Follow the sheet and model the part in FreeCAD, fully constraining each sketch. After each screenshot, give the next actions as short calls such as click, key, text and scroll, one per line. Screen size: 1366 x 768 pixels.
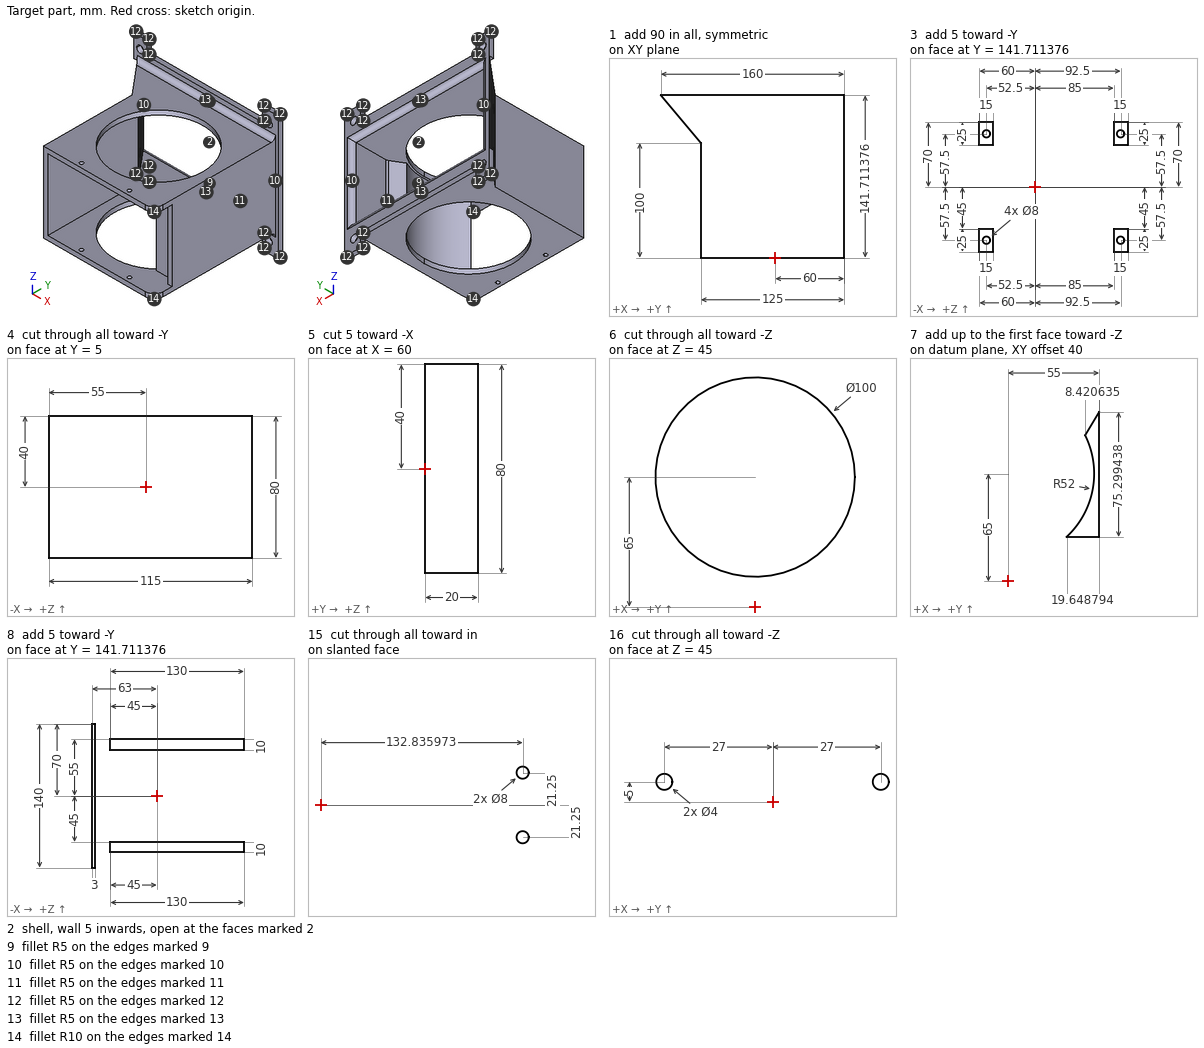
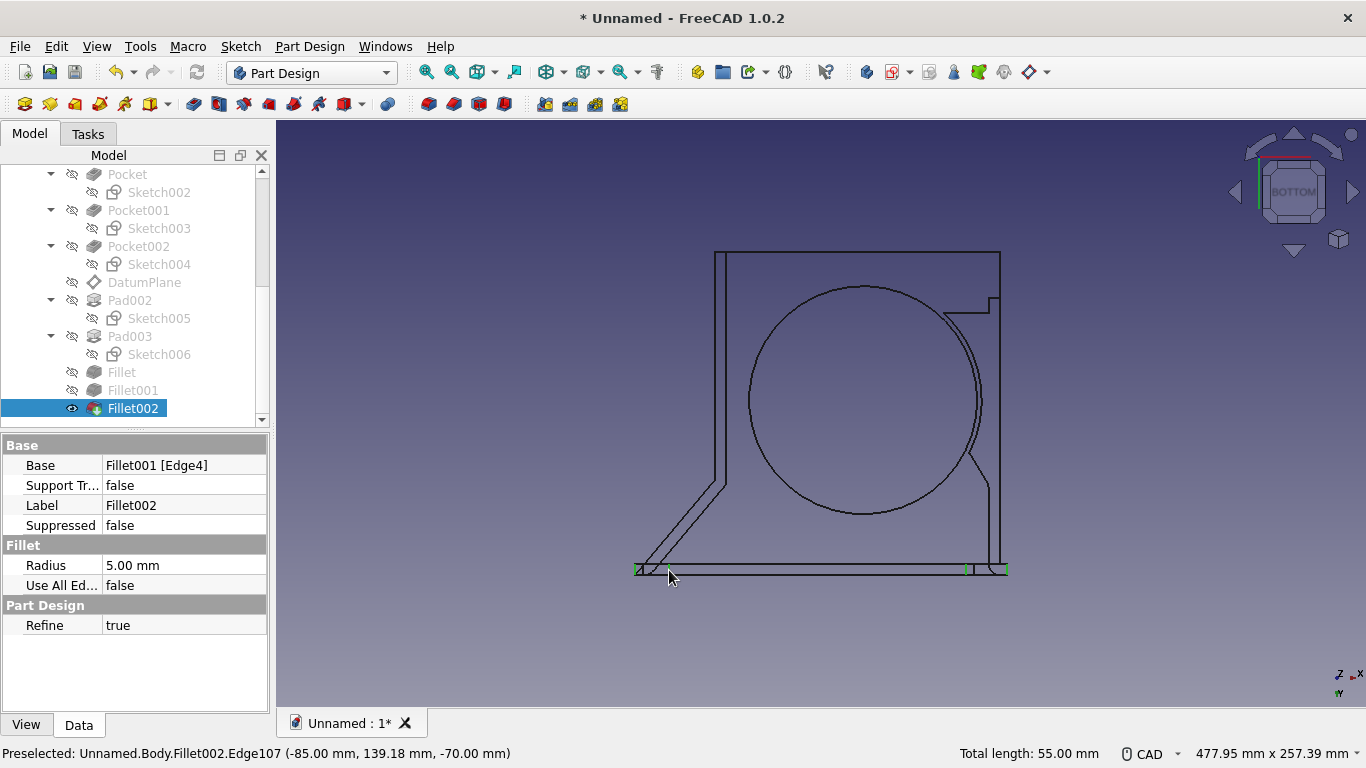
key(4)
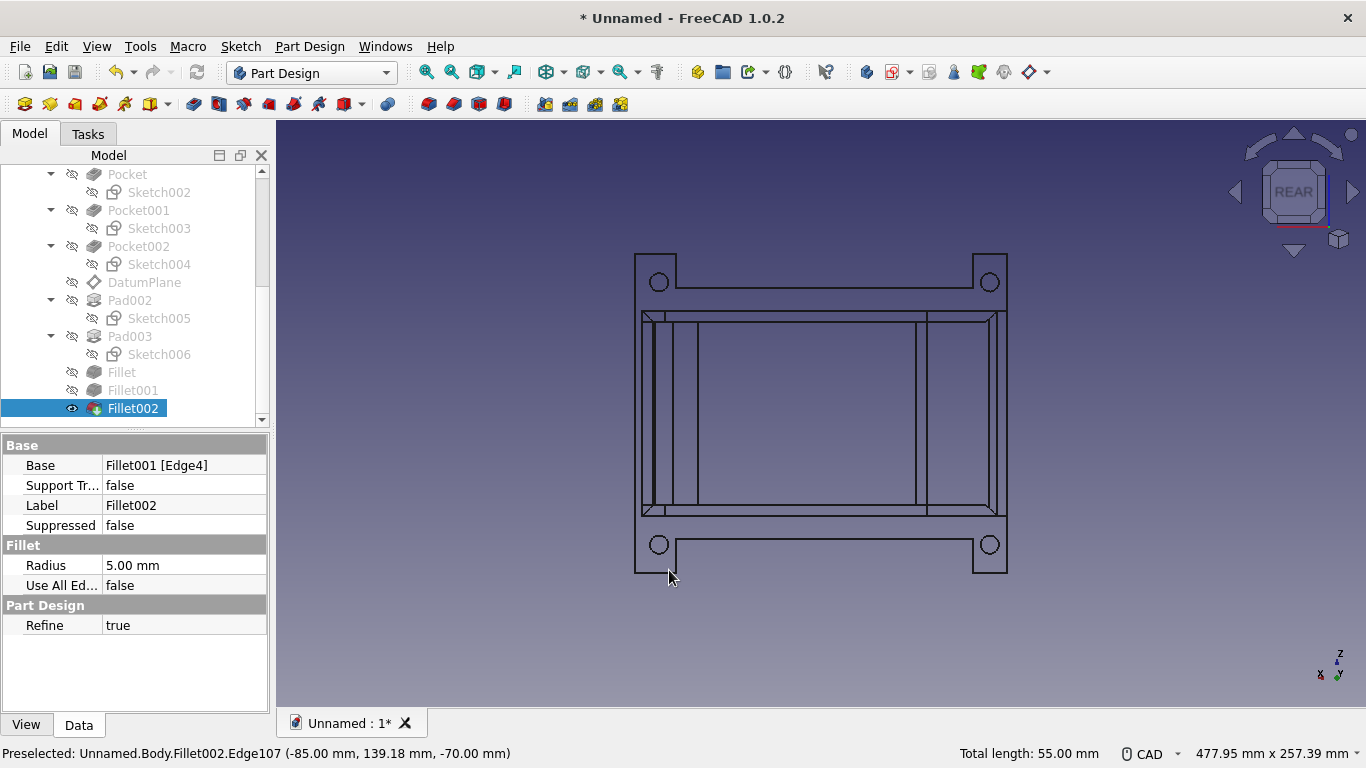
scroll(973, 287, up, 7)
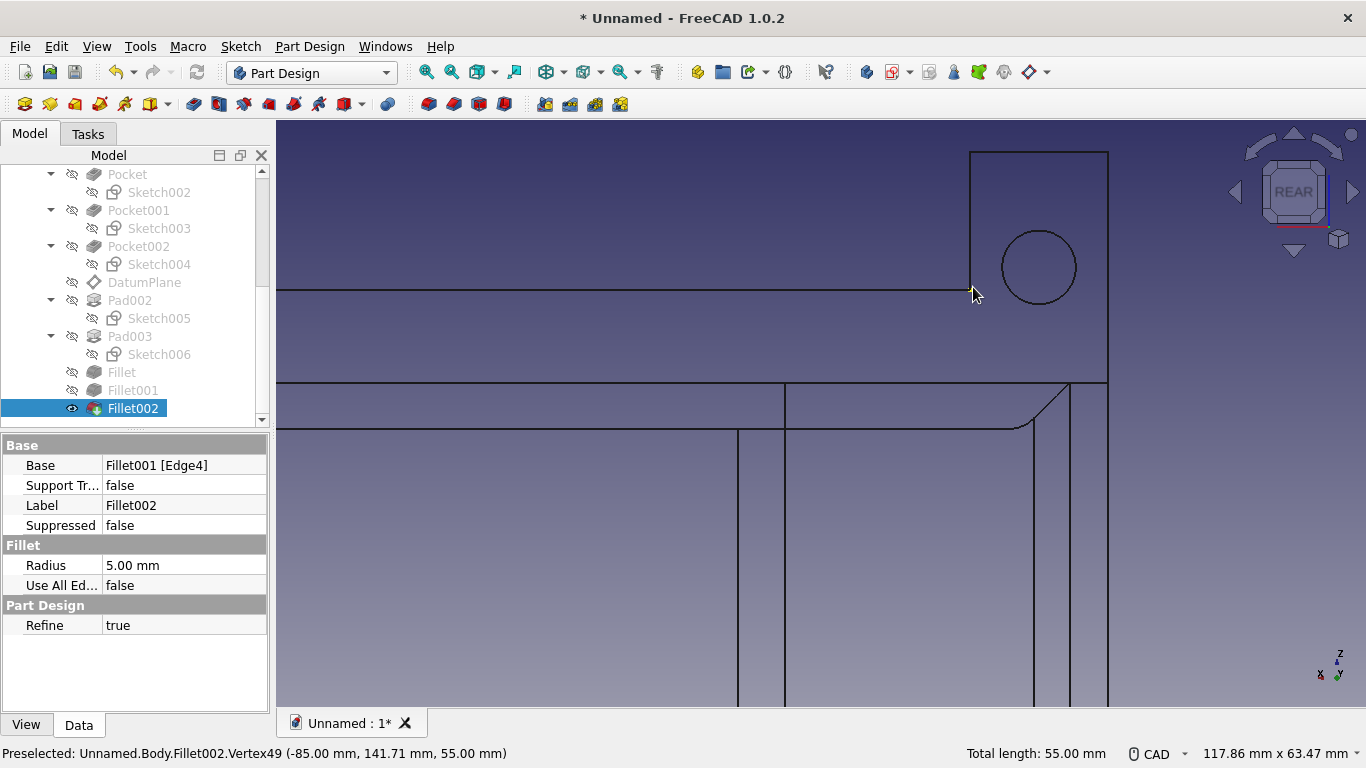
key(v)
key(f)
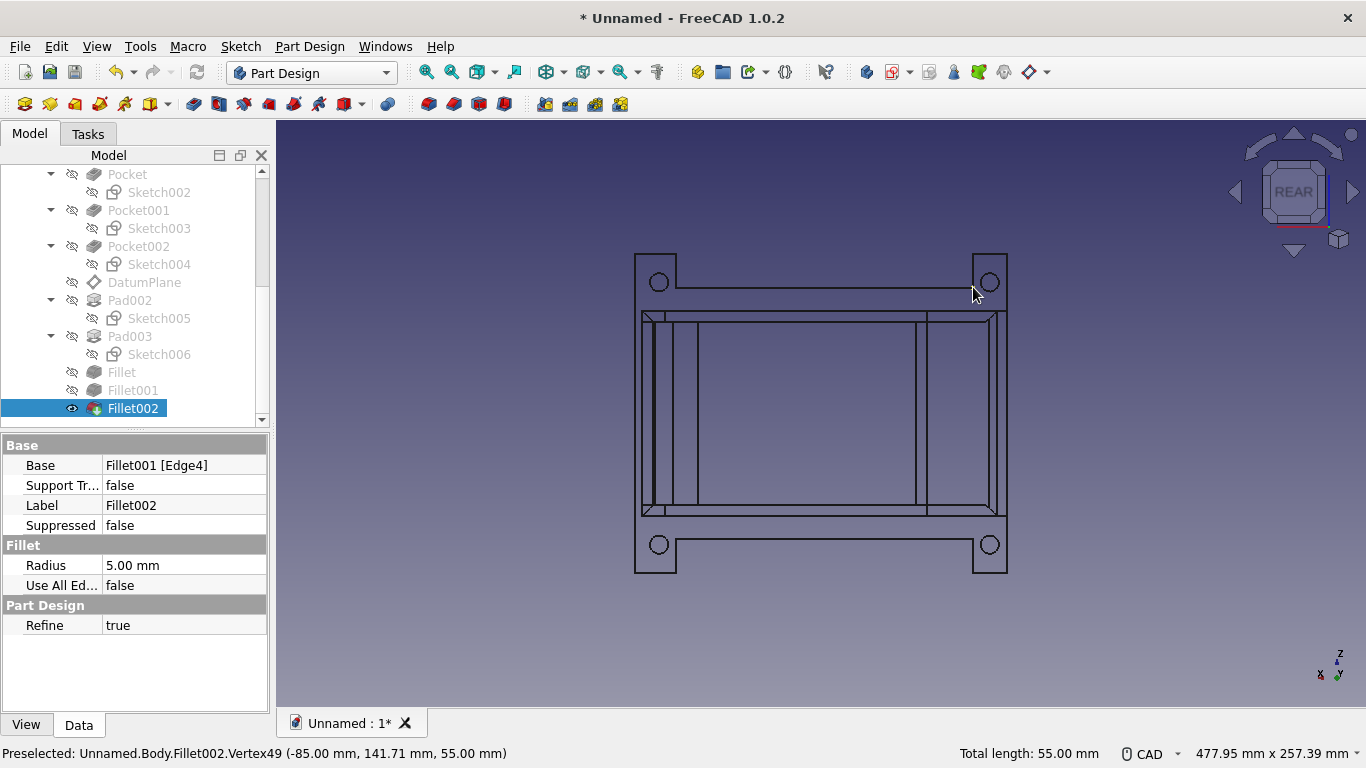
key(6)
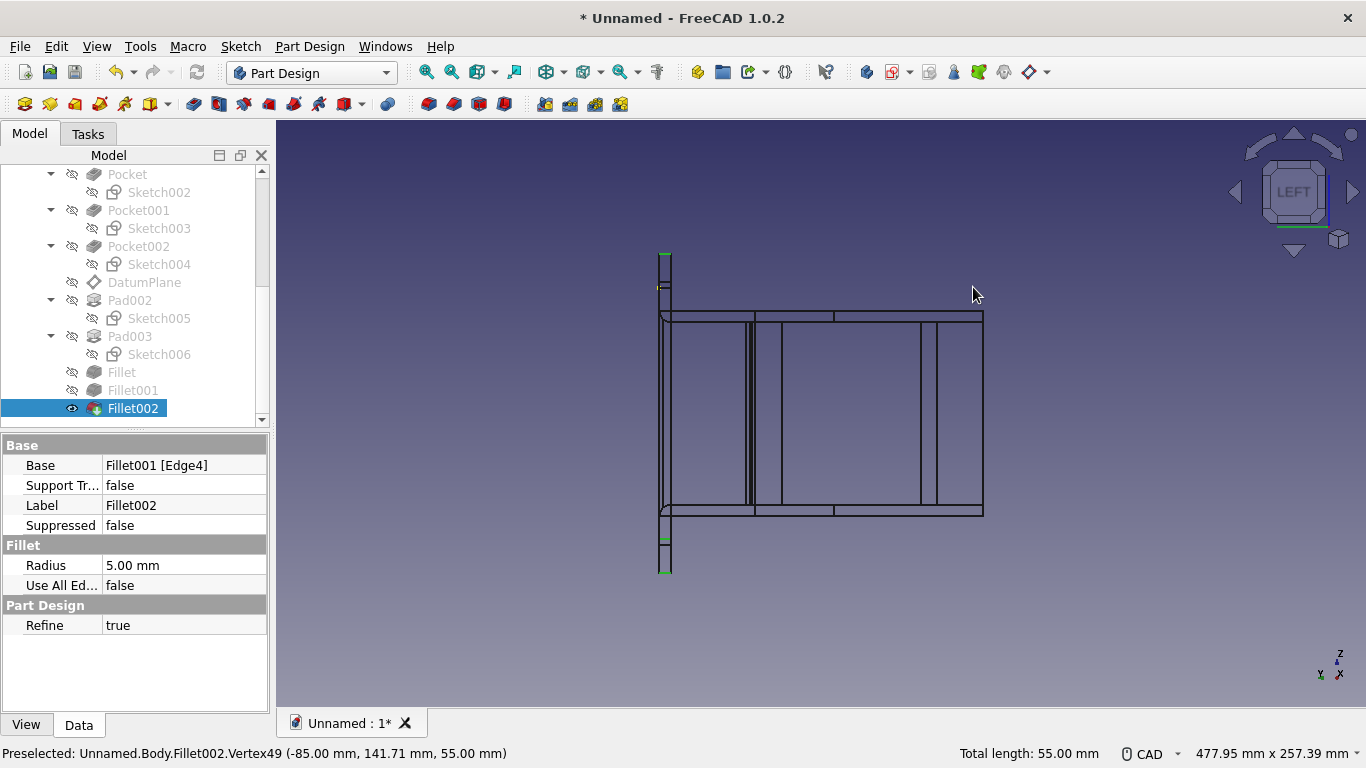
scroll(665, 287, up, 7)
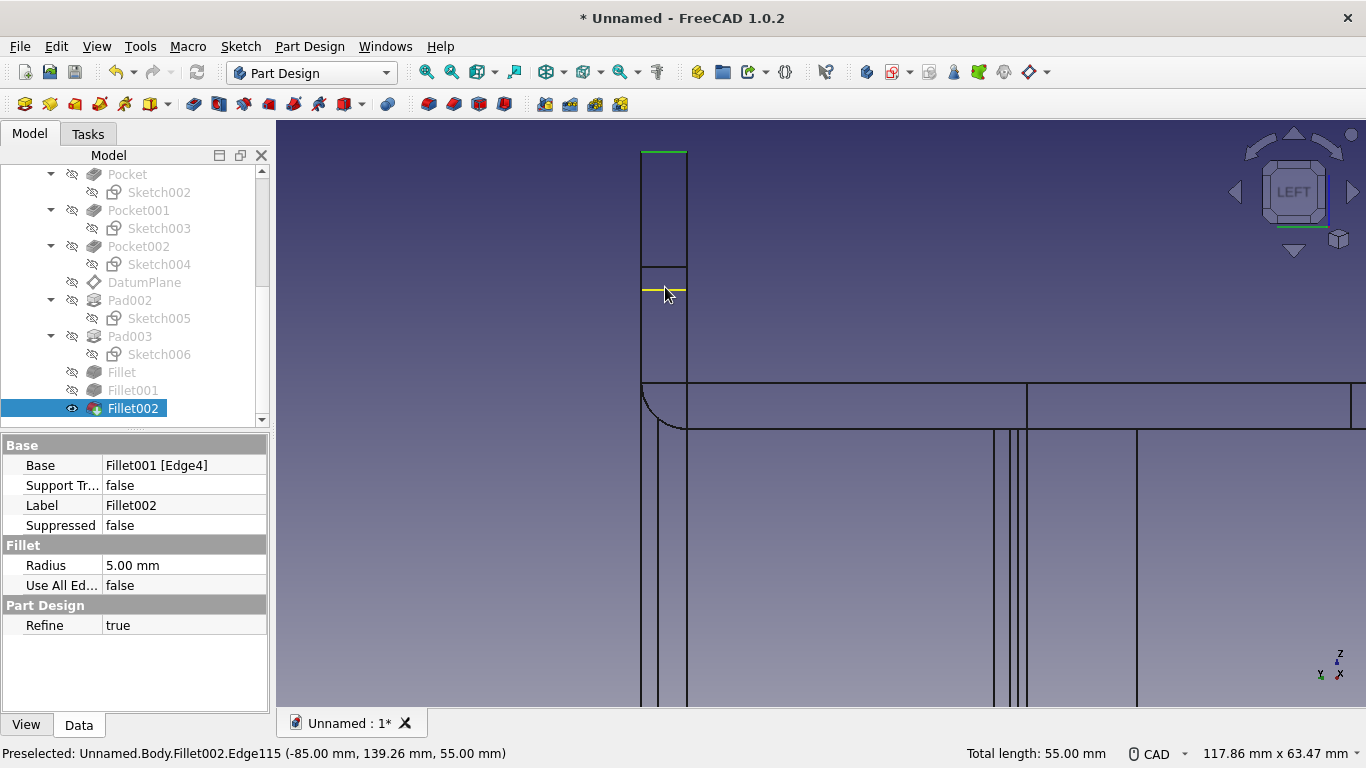
click(664, 289, ctrl)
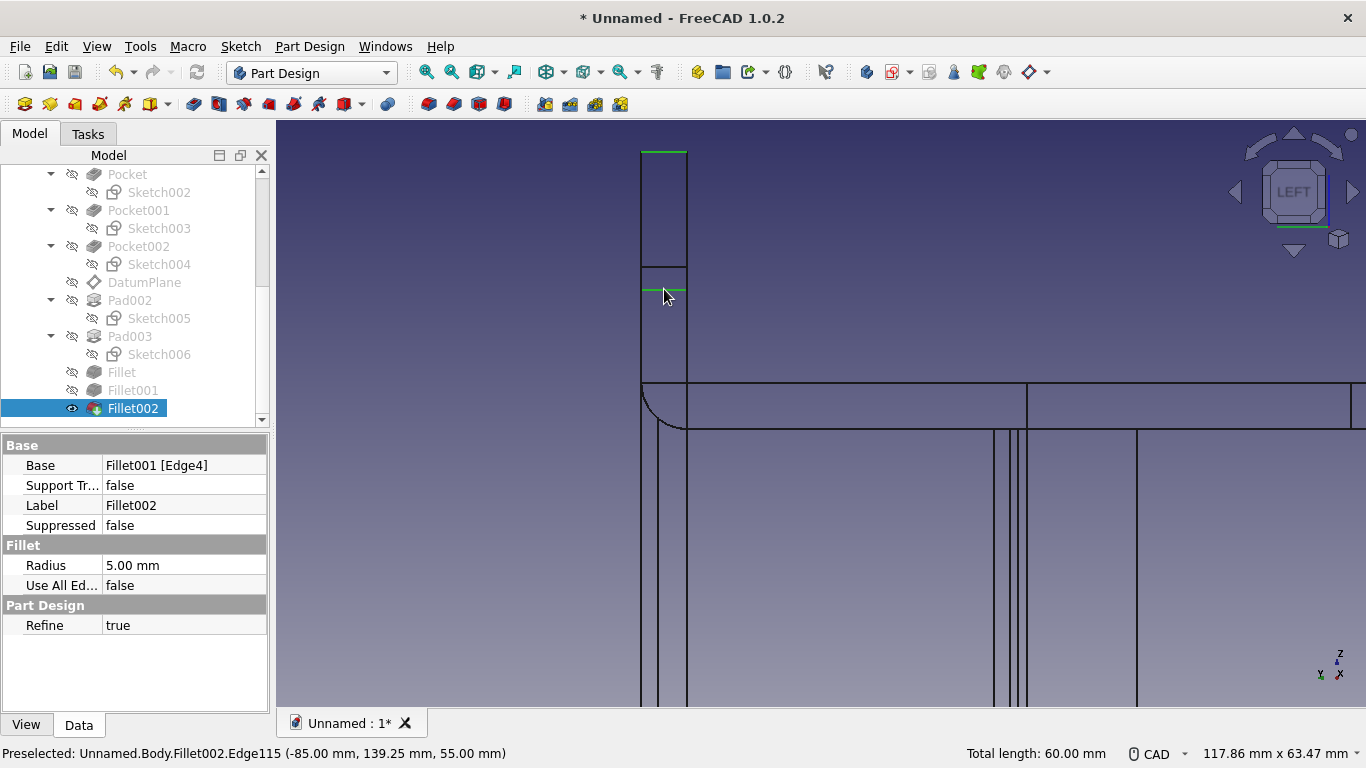
key(v)
key(1)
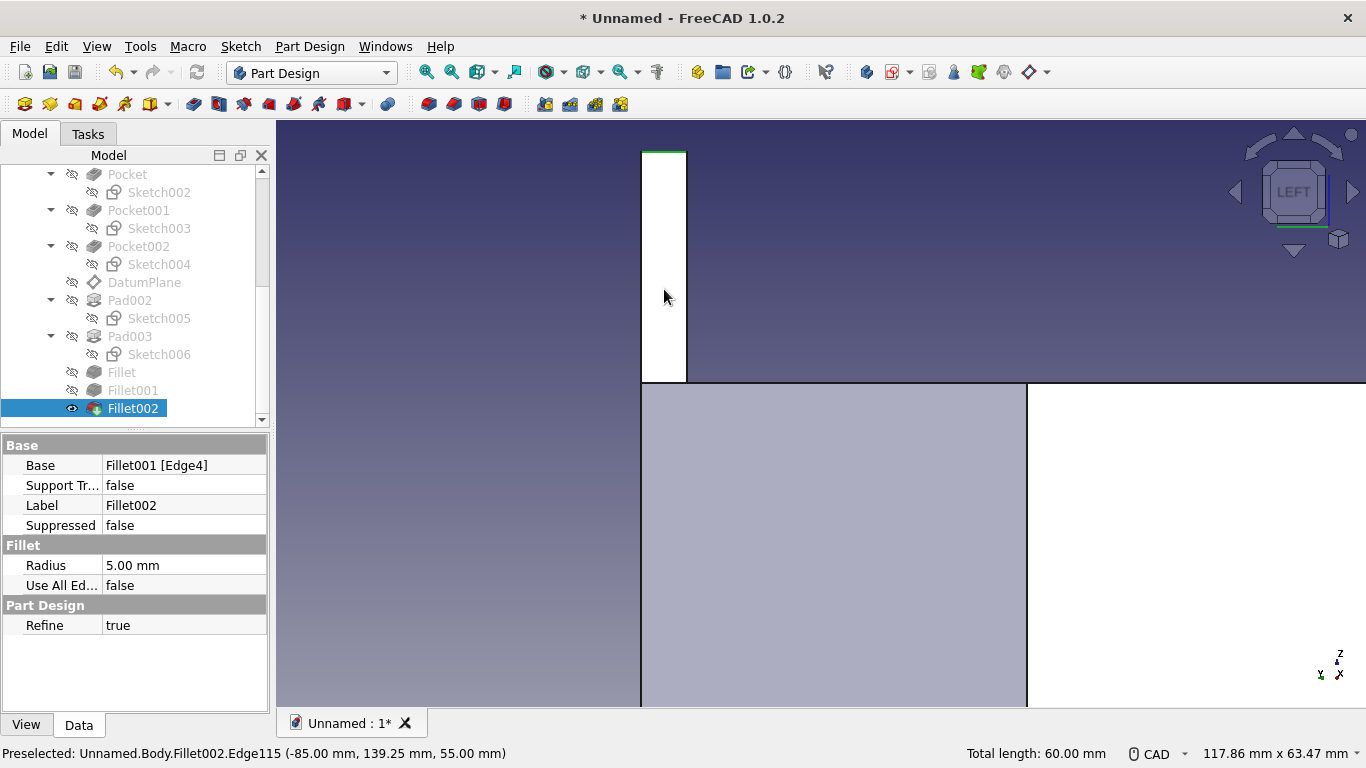
click(429, 104)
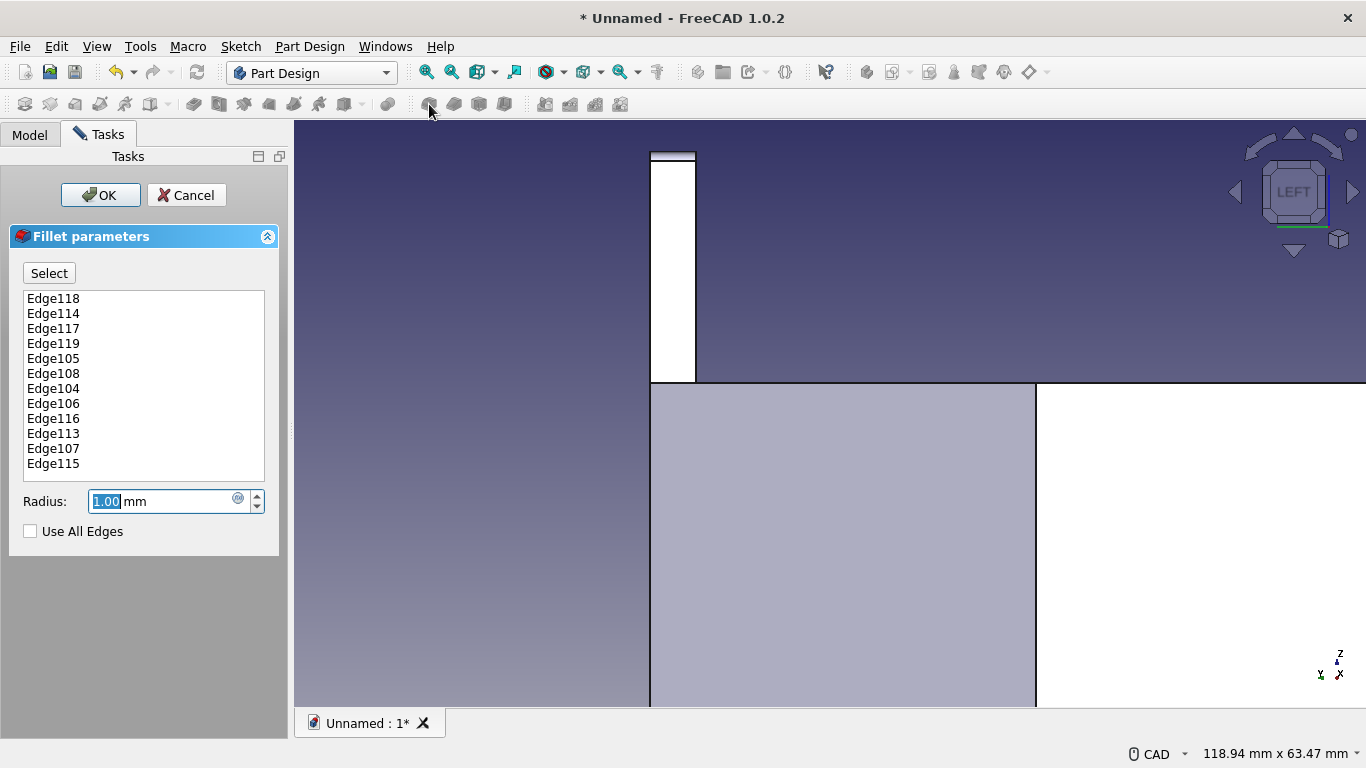
text(5)
key(Tab)